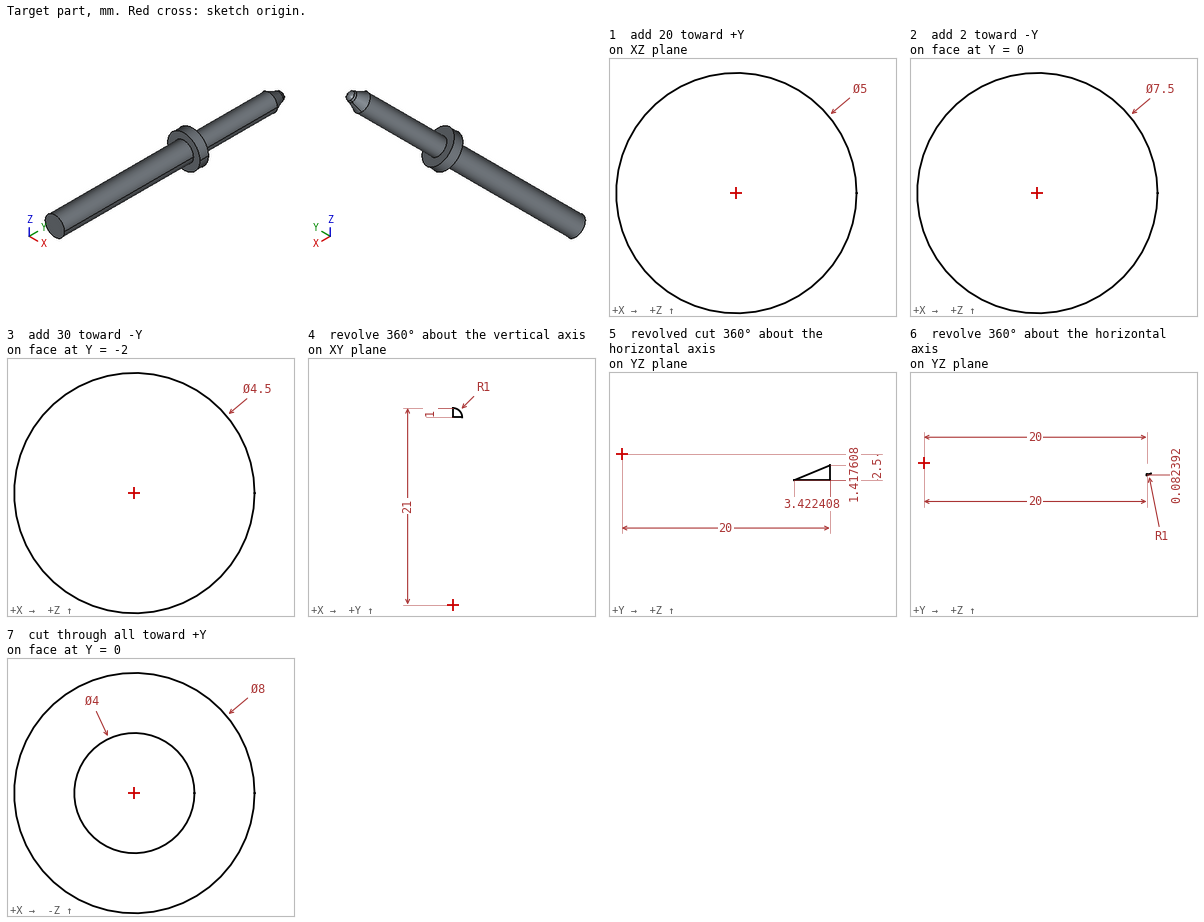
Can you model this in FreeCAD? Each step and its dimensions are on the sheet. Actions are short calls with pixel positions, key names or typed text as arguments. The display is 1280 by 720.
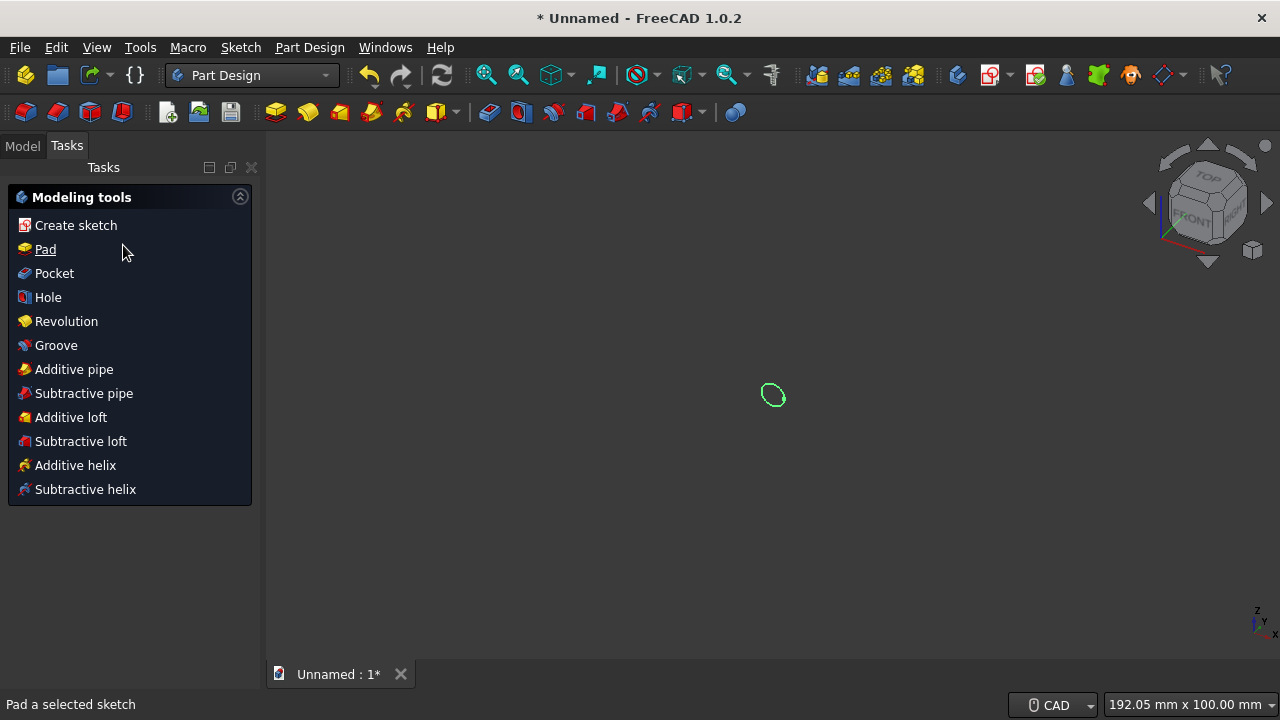
click(276, 112)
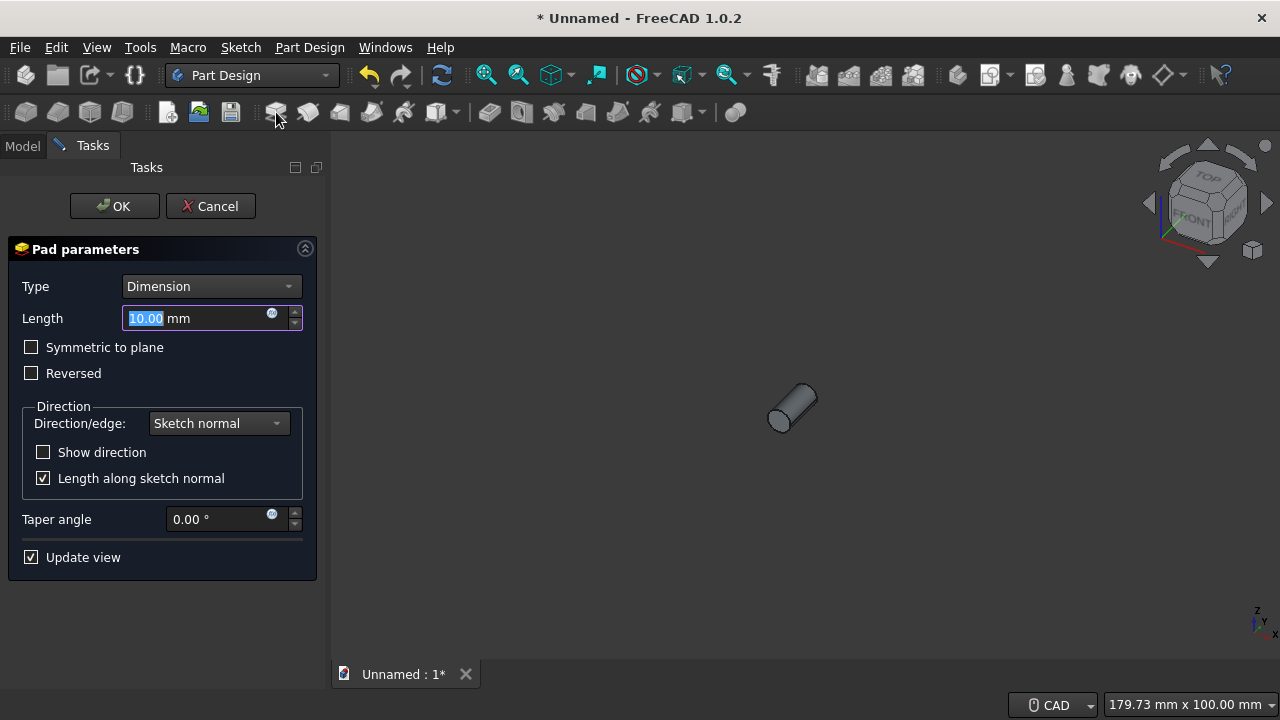
text(20)
key(Tab)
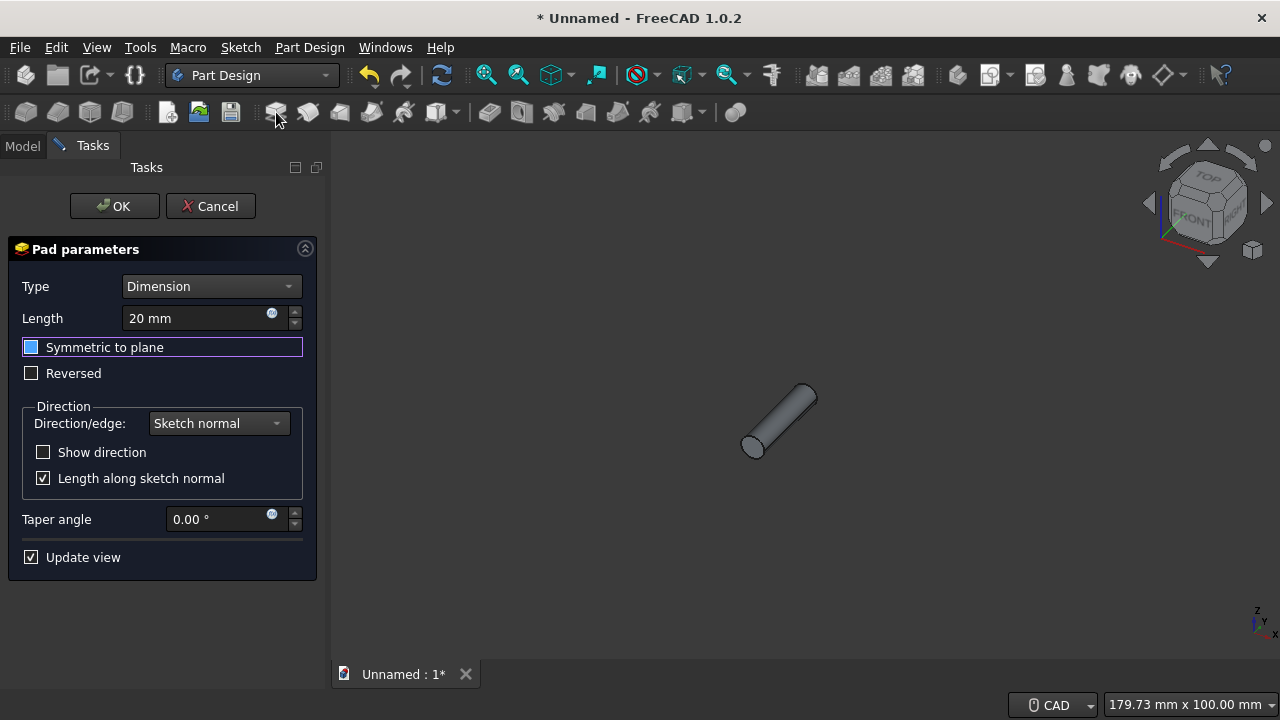
click(30, 373)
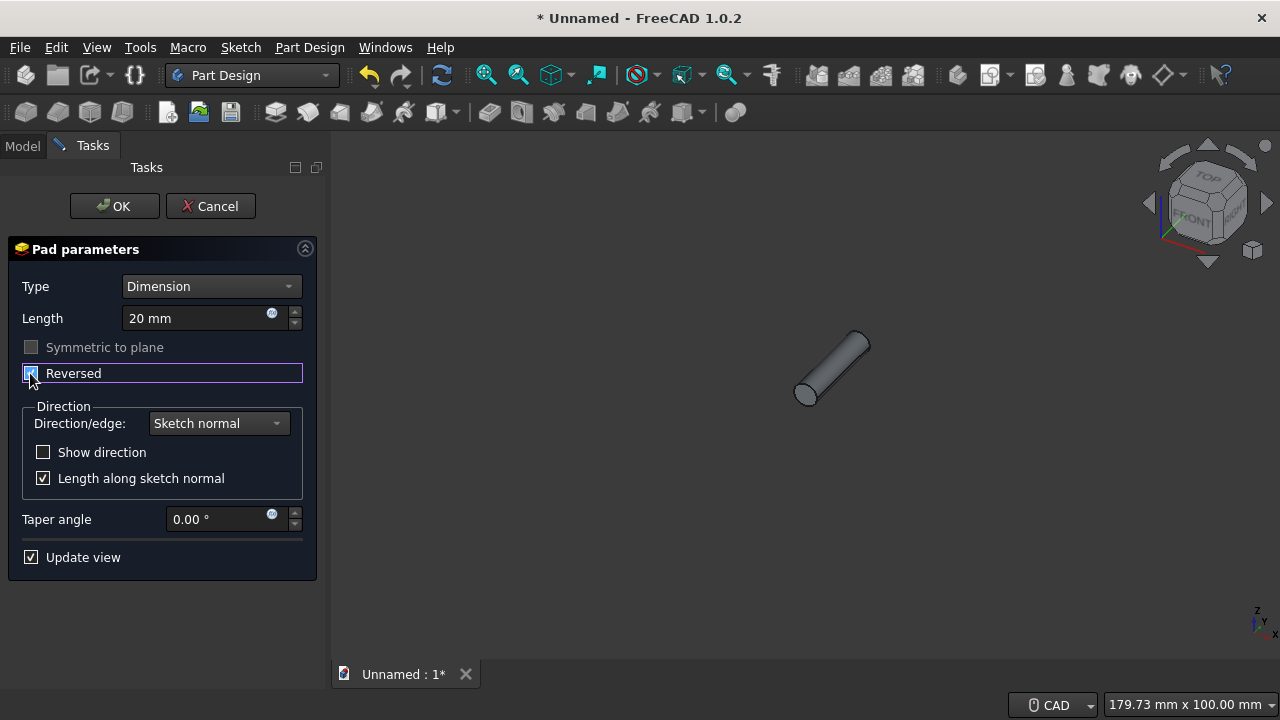
click(115, 206)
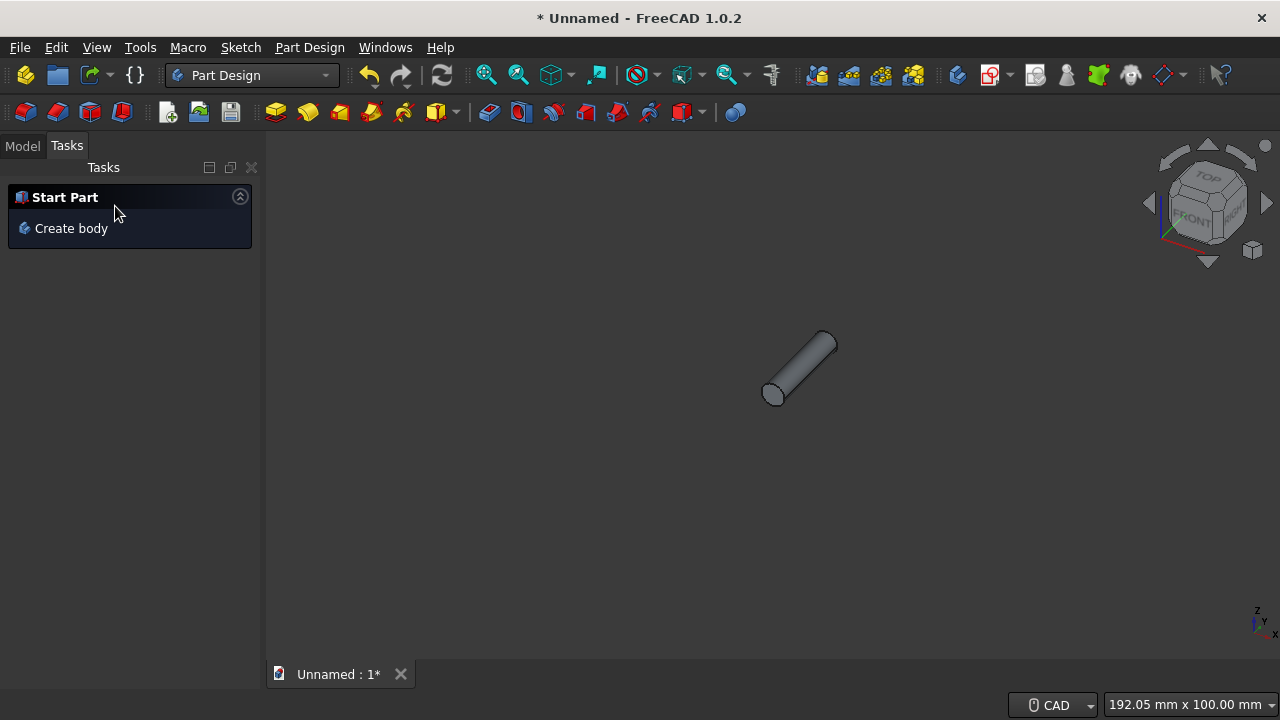
click(488, 76)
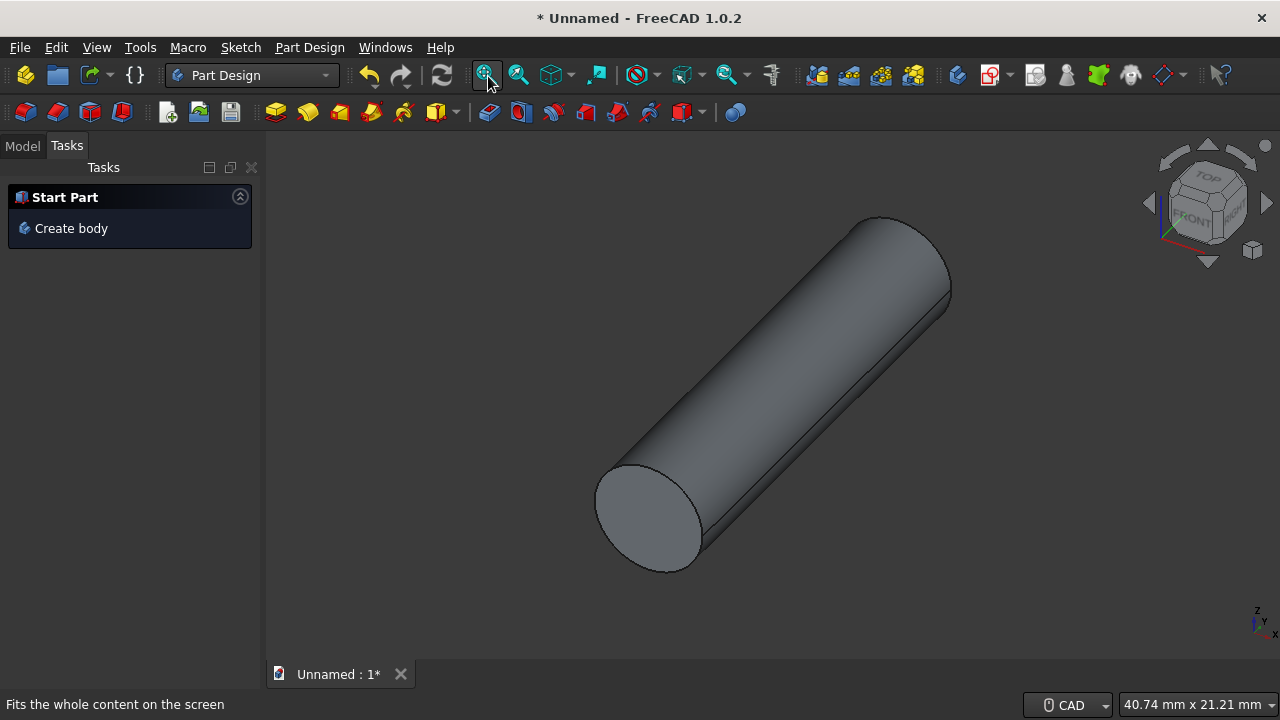
click(649, 518)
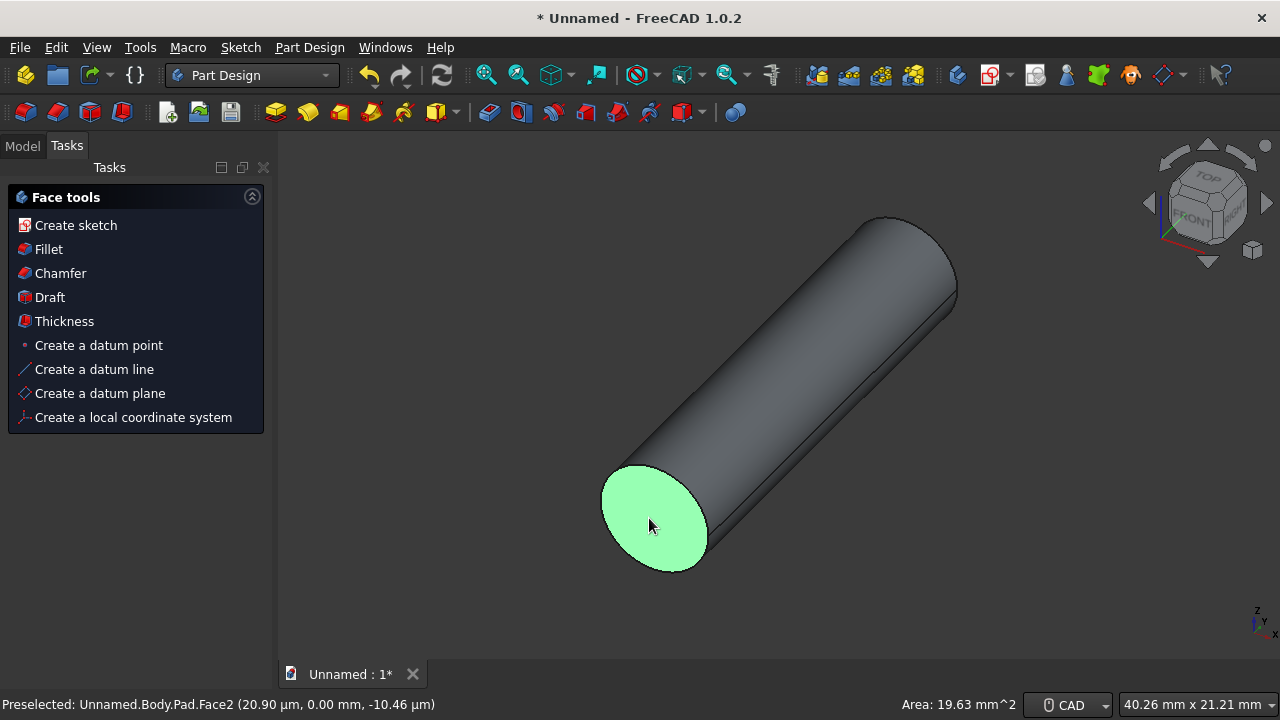
click(990, 76)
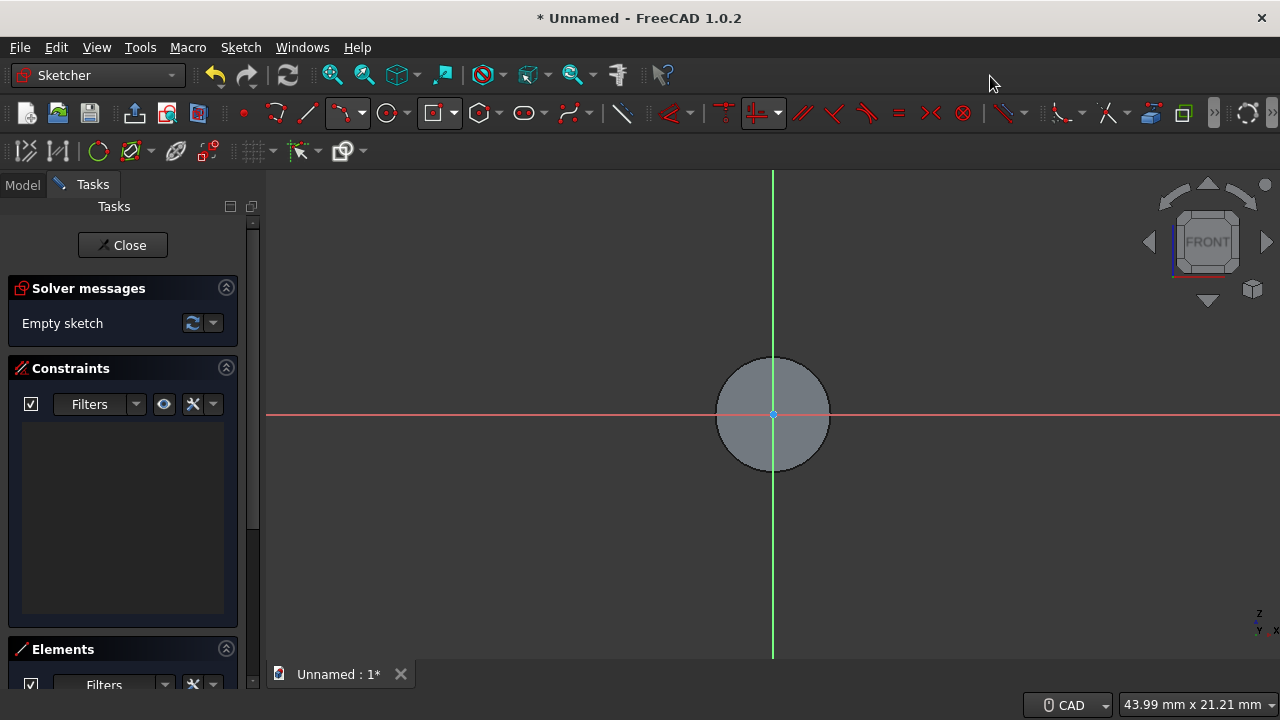
scroll(856, 415, up, 3)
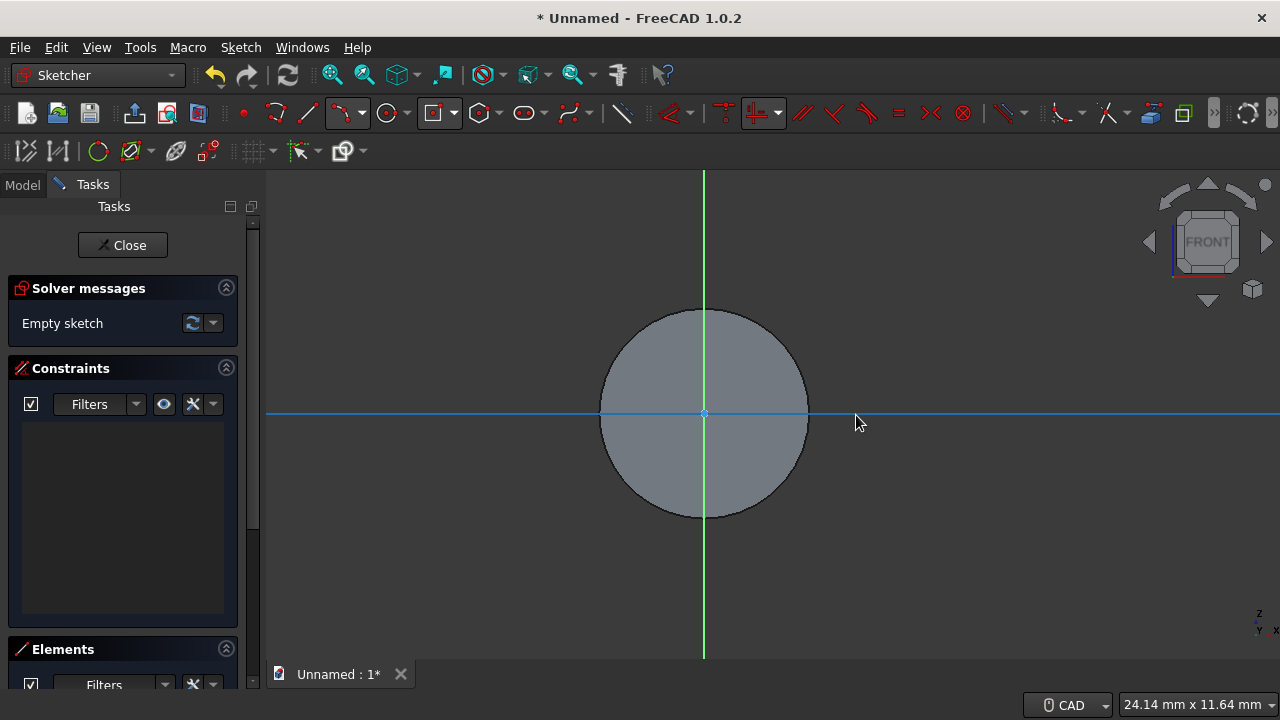
click(388, 114)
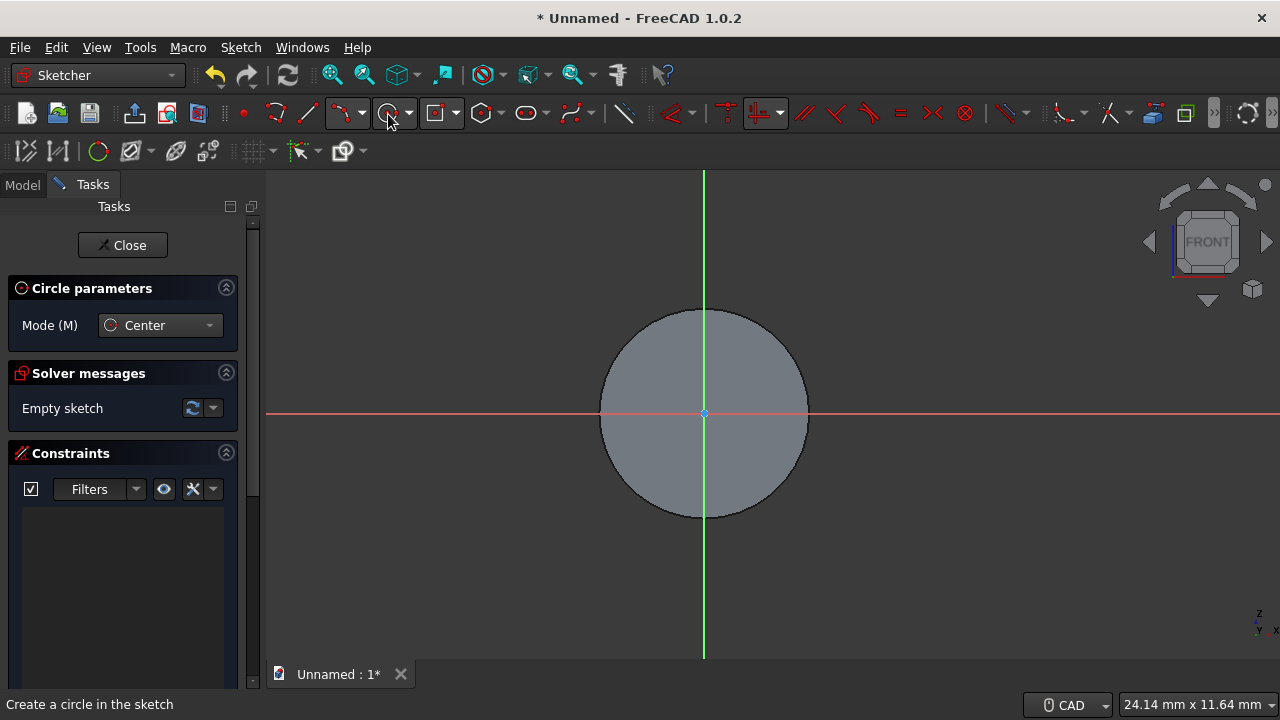
click(704, 414)
click(816, 302)
key(Escape)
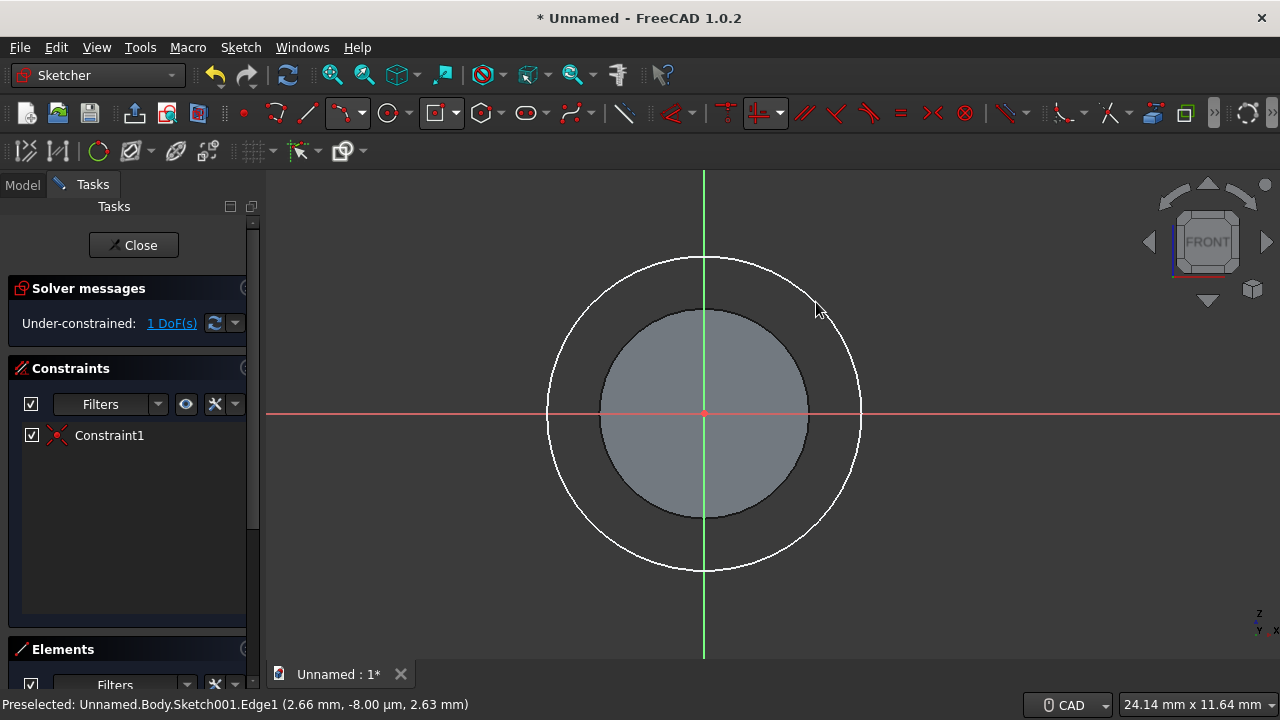
click(672, 114)